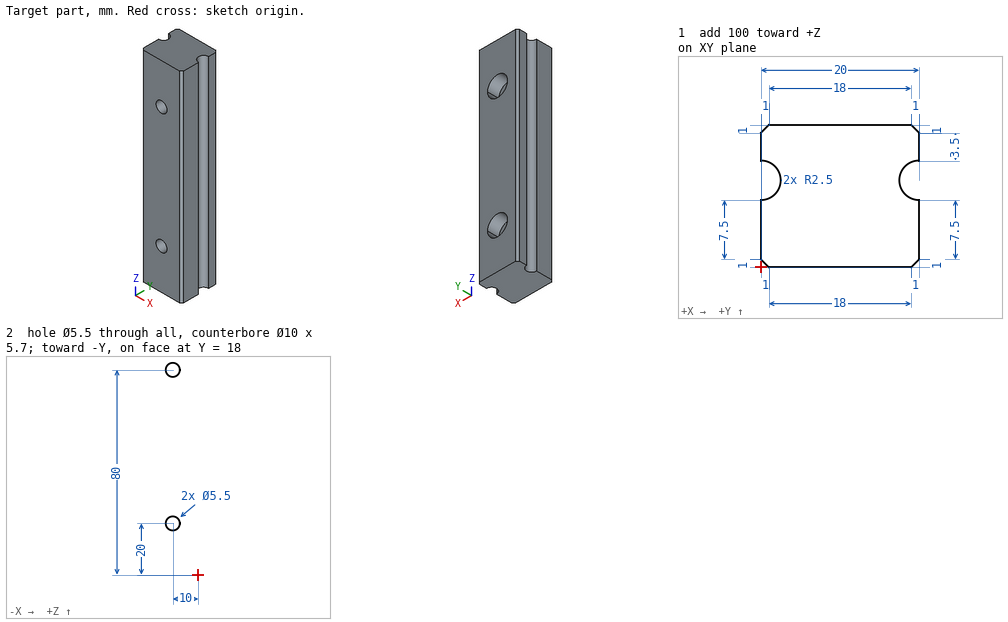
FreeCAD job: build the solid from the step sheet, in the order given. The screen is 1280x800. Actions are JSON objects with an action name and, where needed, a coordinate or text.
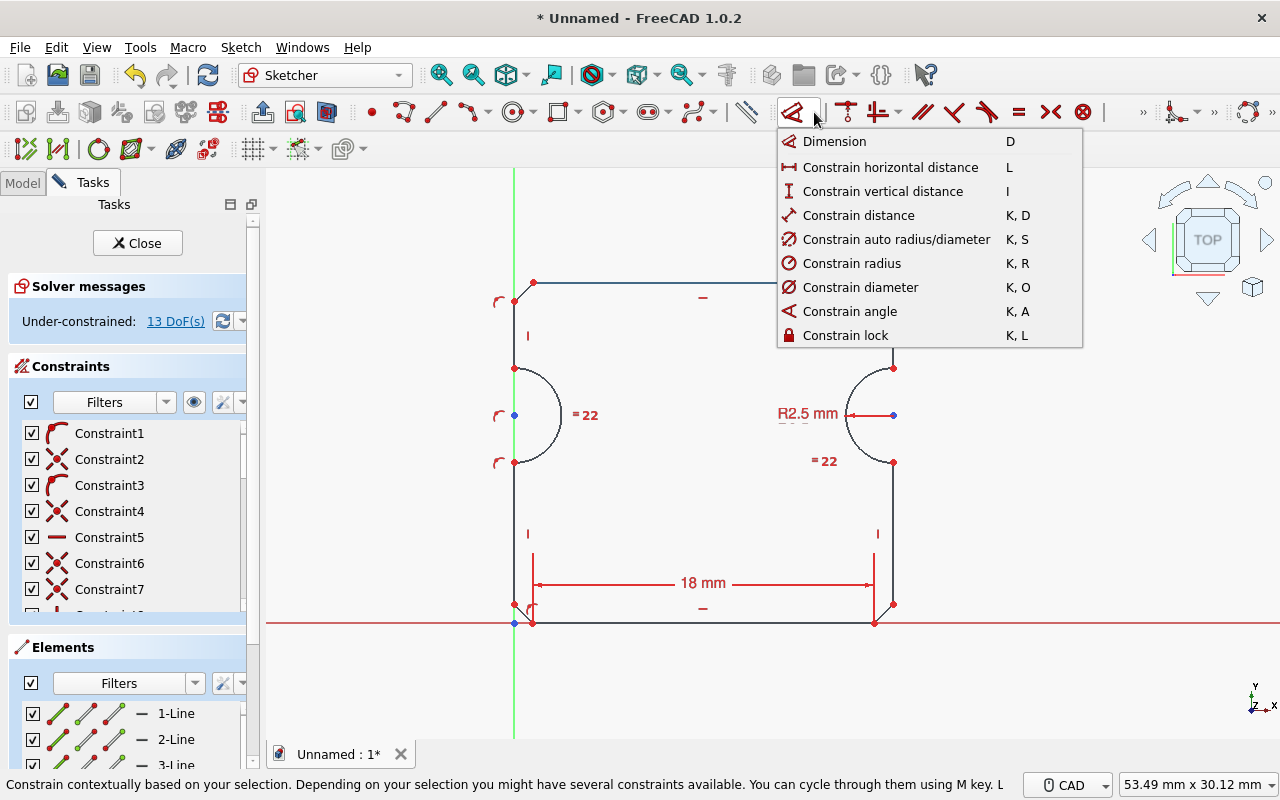
{"action": "left_click", "coordinate": [930, 167]}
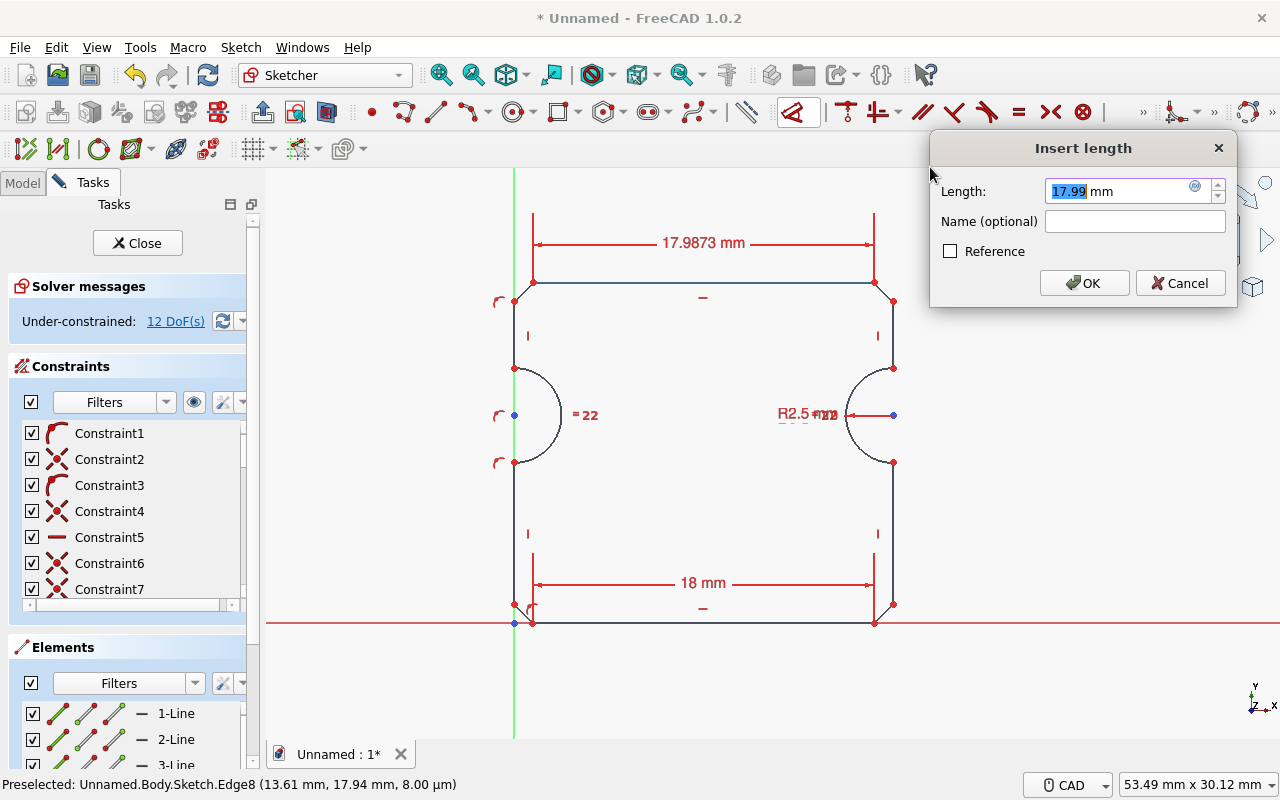
{"action": "type", "text": "18"}
{"action": "key", "text": "Return"}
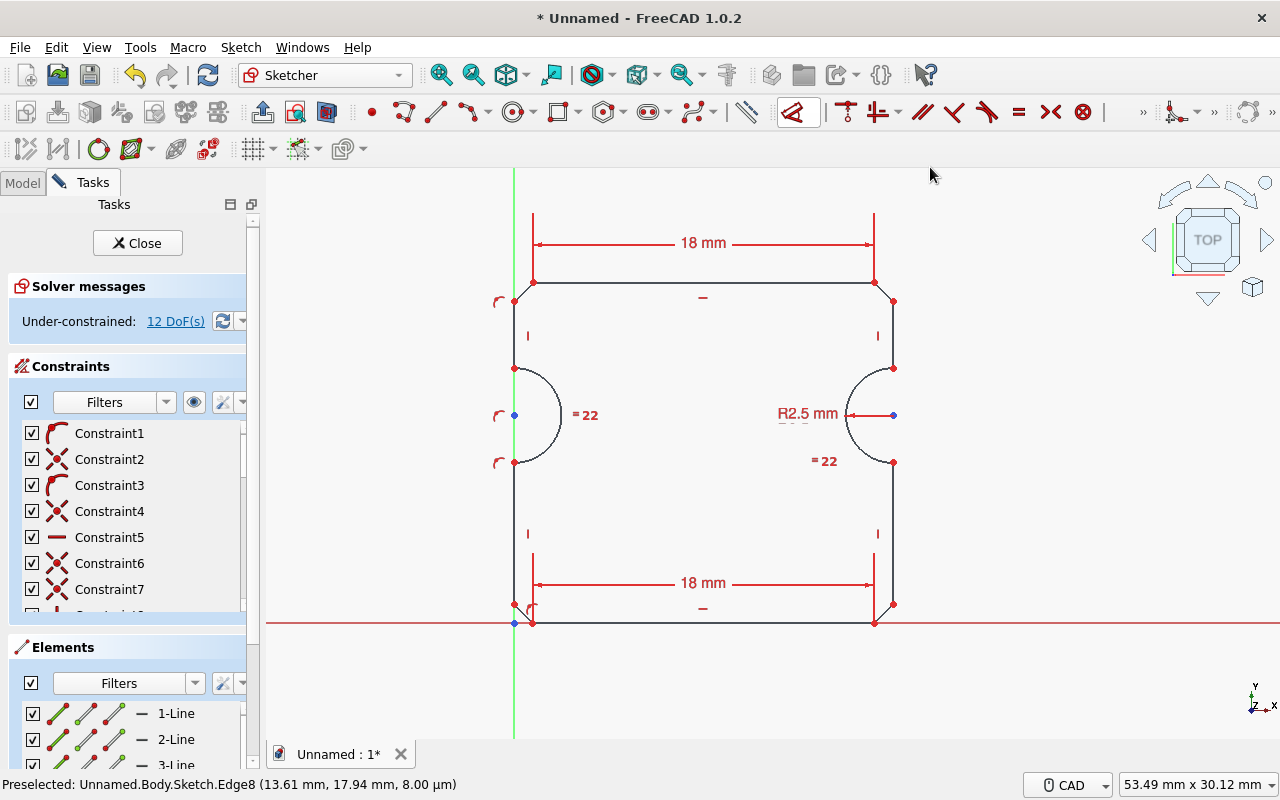
{"action": "scroll", "coordinate": [514, 605], "scroll_direction": "up", "scroll_amount": 4}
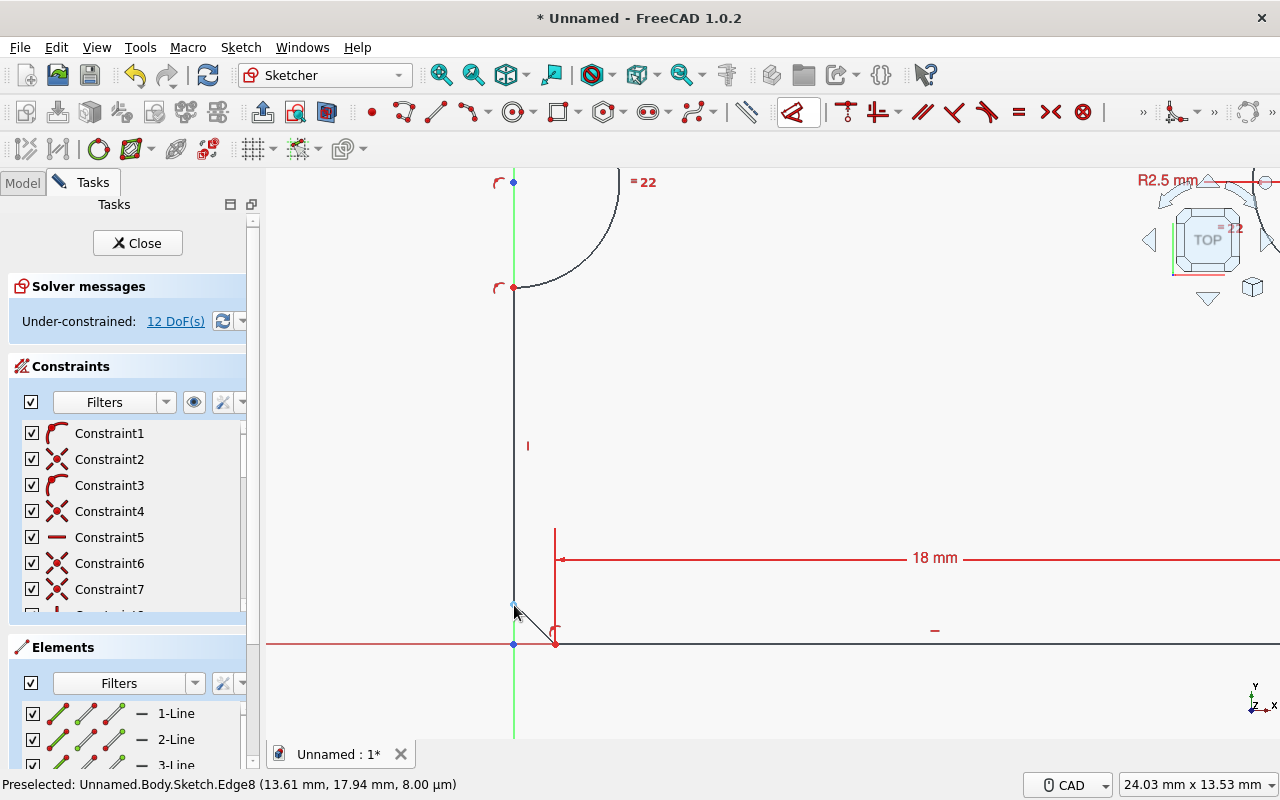
{"action": "left_click", "coordinate": [514, 604]}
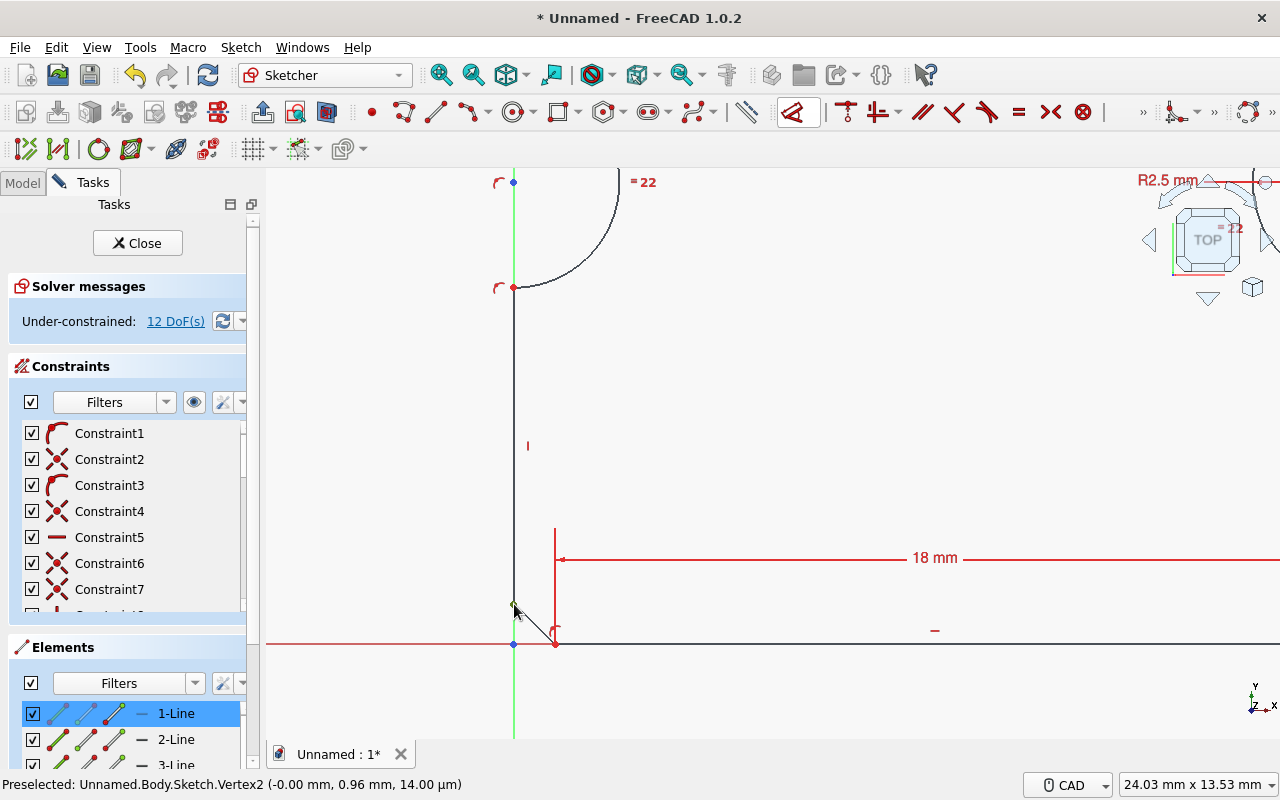
{"action": "left_click", "coordinate": [814, 112]}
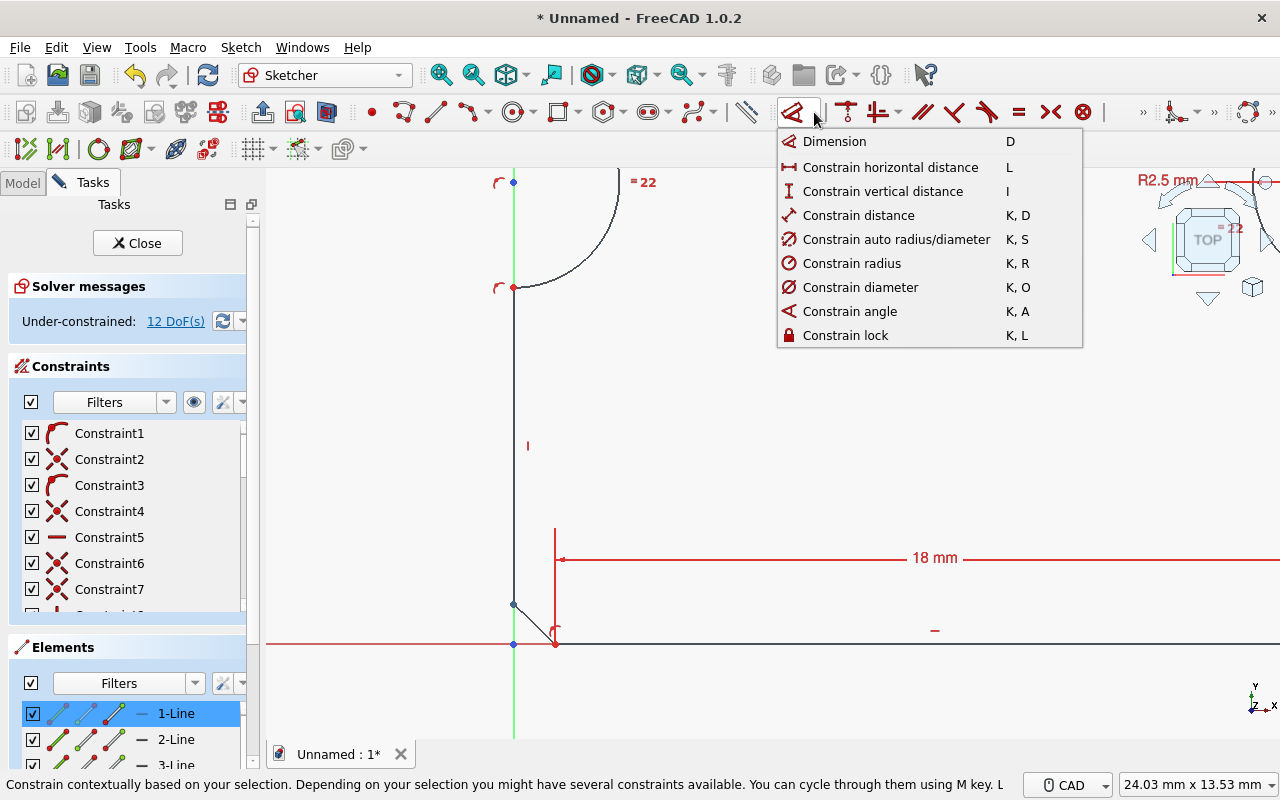
{"action": "left_click", "coordinate": [930, 191]}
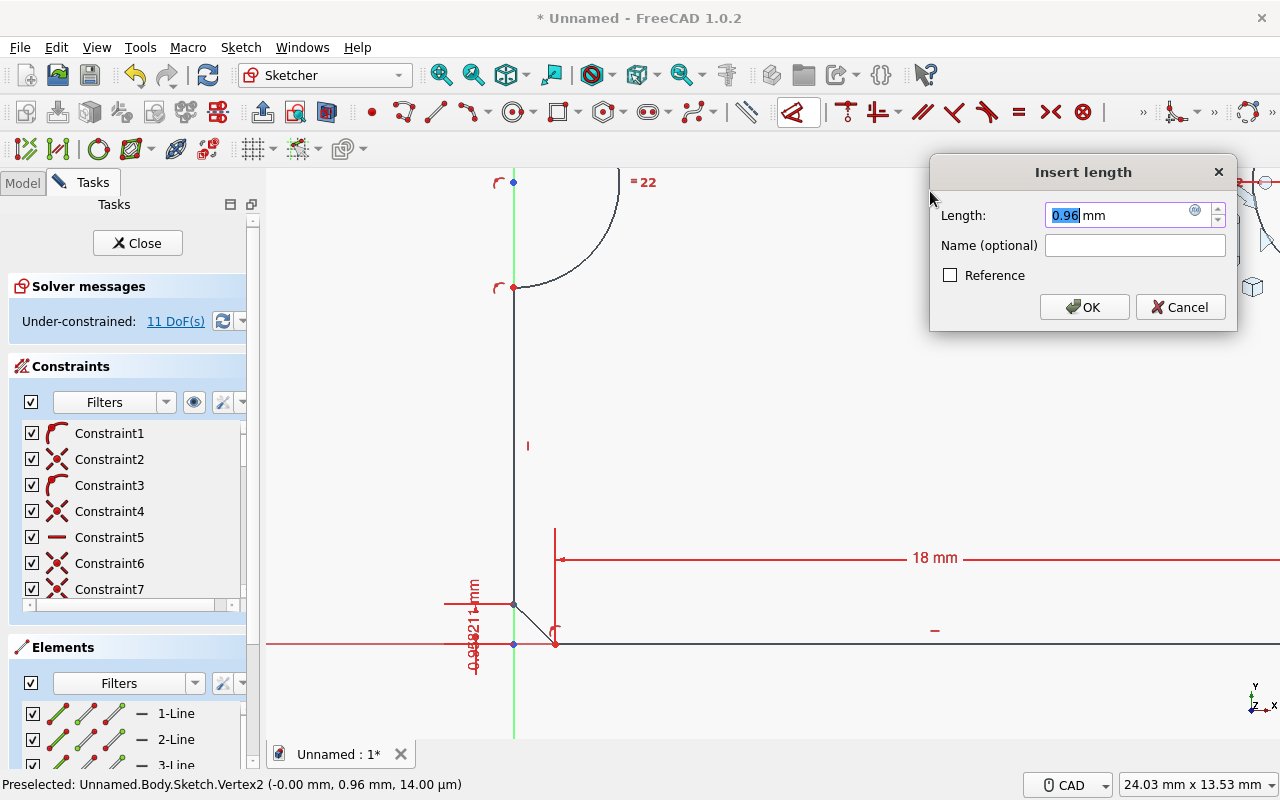
{"action": "type", "text": "1"}
{"action": "key", "text": "Return"}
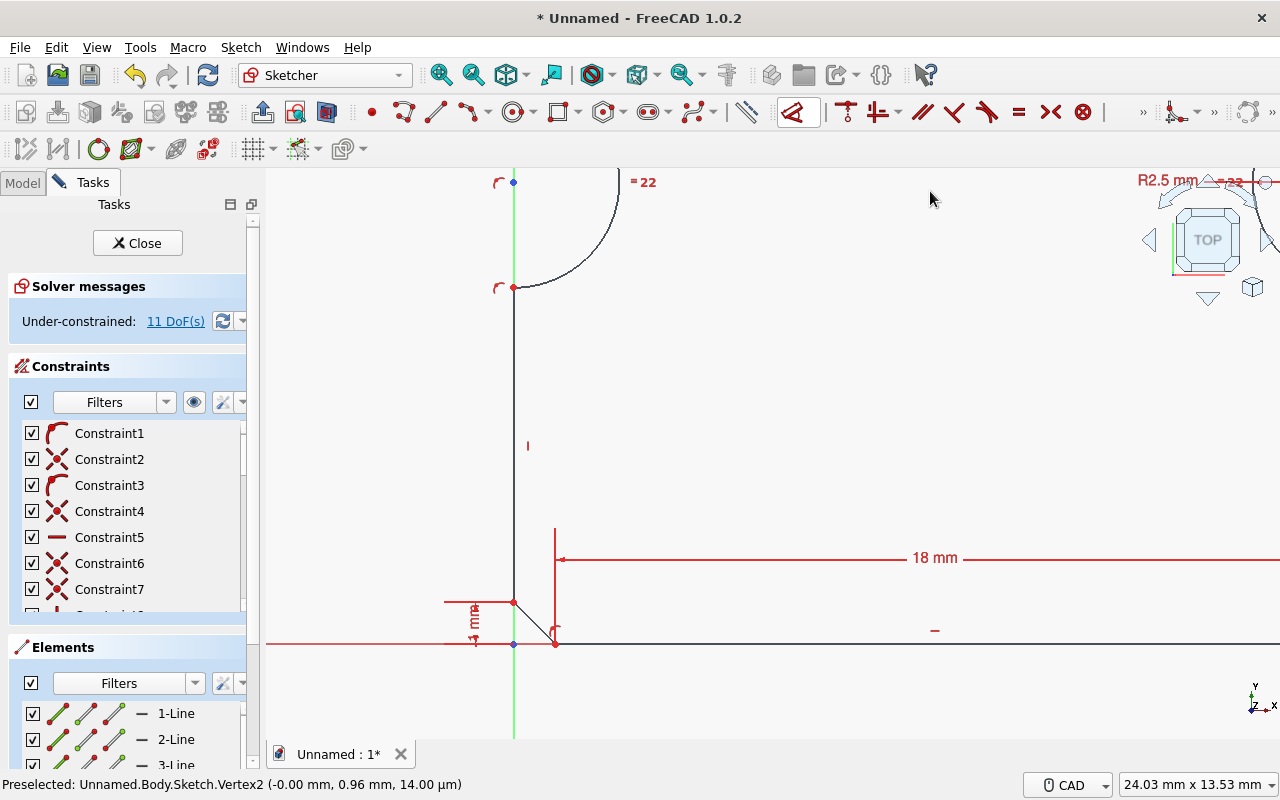
{"action": "left_click", "coordinate": [555, 644]}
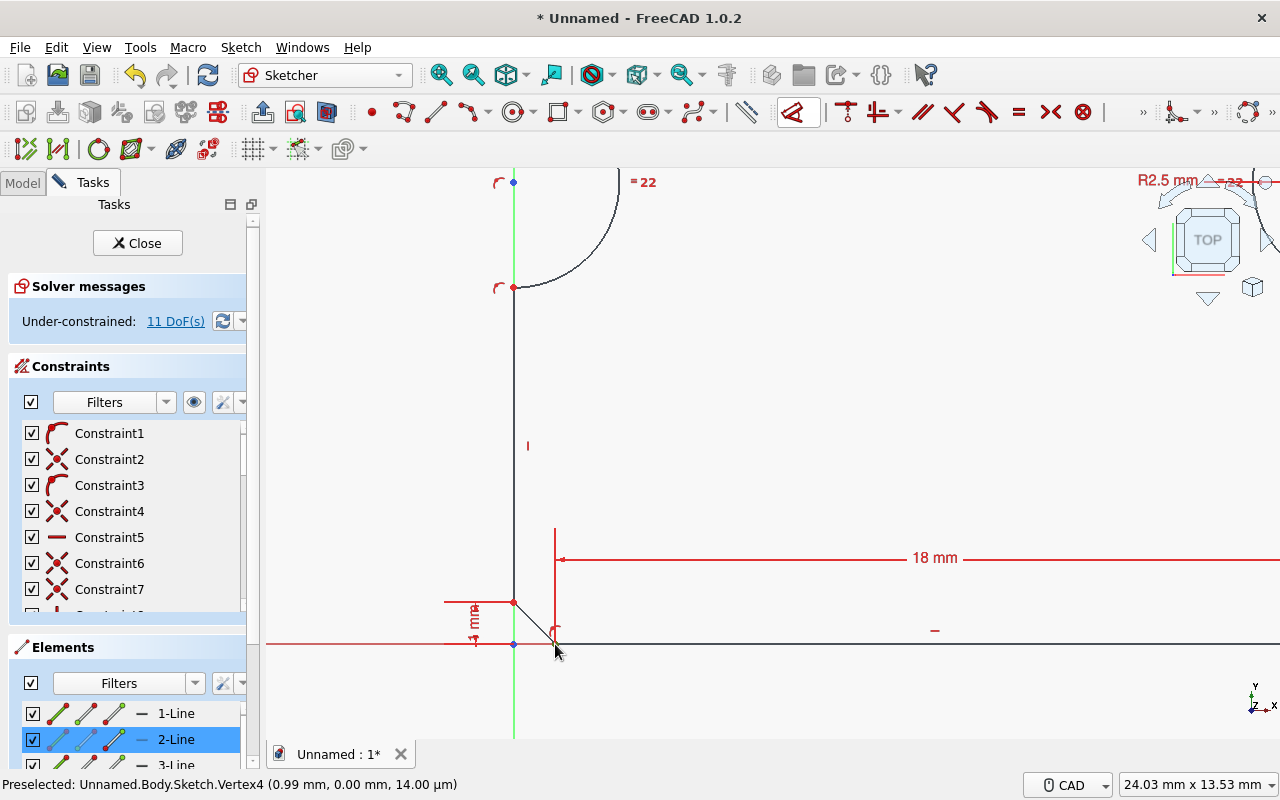
{"action": "left_click", "coordinate": [814, 112]}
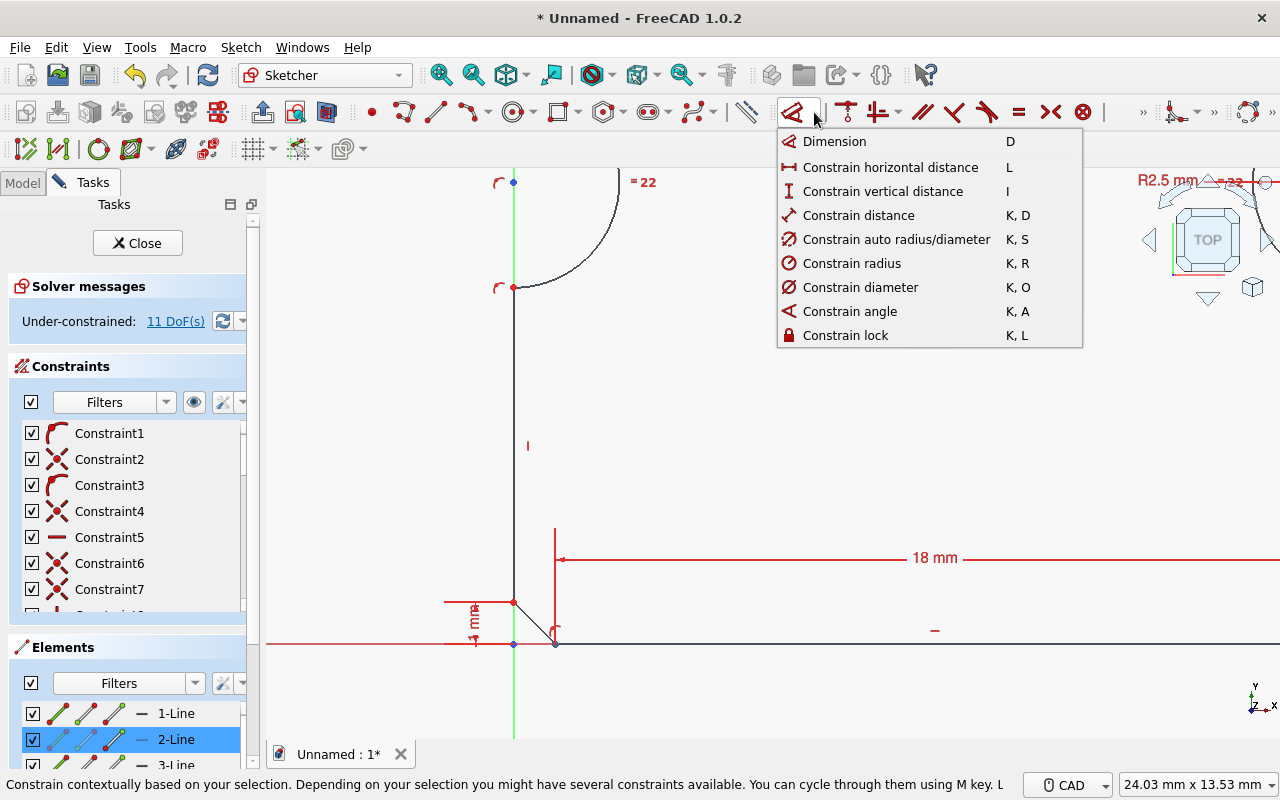
{"action": "left_click", "coordinate": [930, 167]}